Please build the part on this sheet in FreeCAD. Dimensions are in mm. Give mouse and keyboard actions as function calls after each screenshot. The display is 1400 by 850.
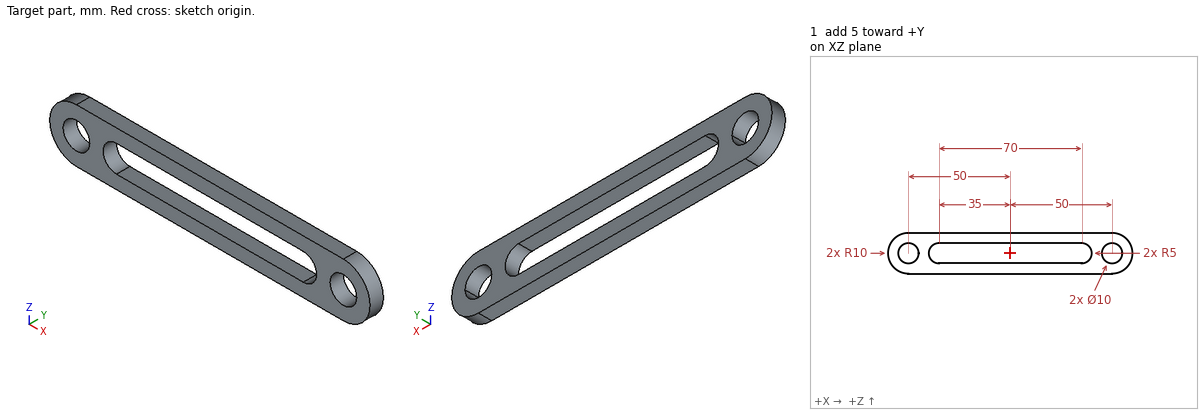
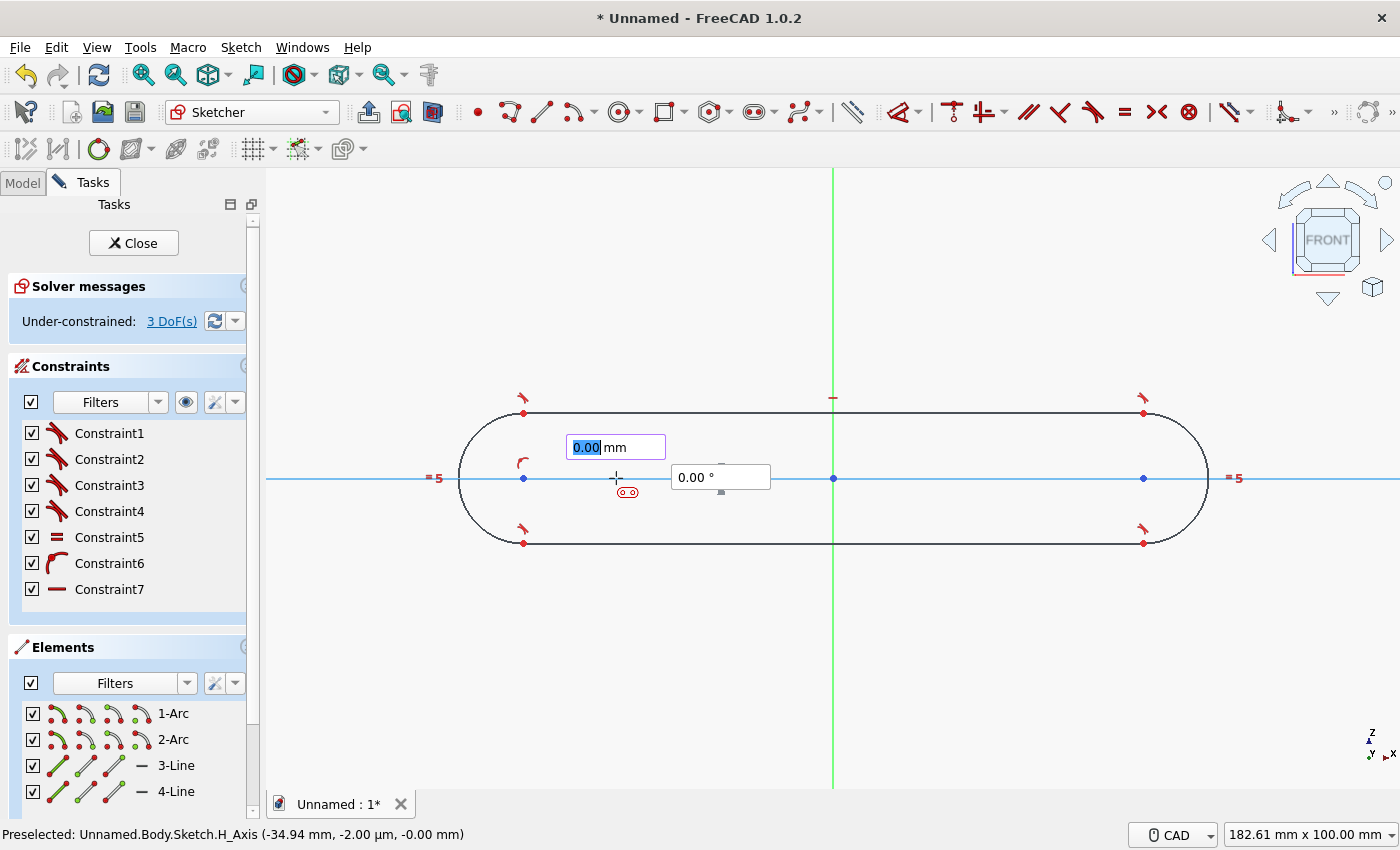
click(1050, 470)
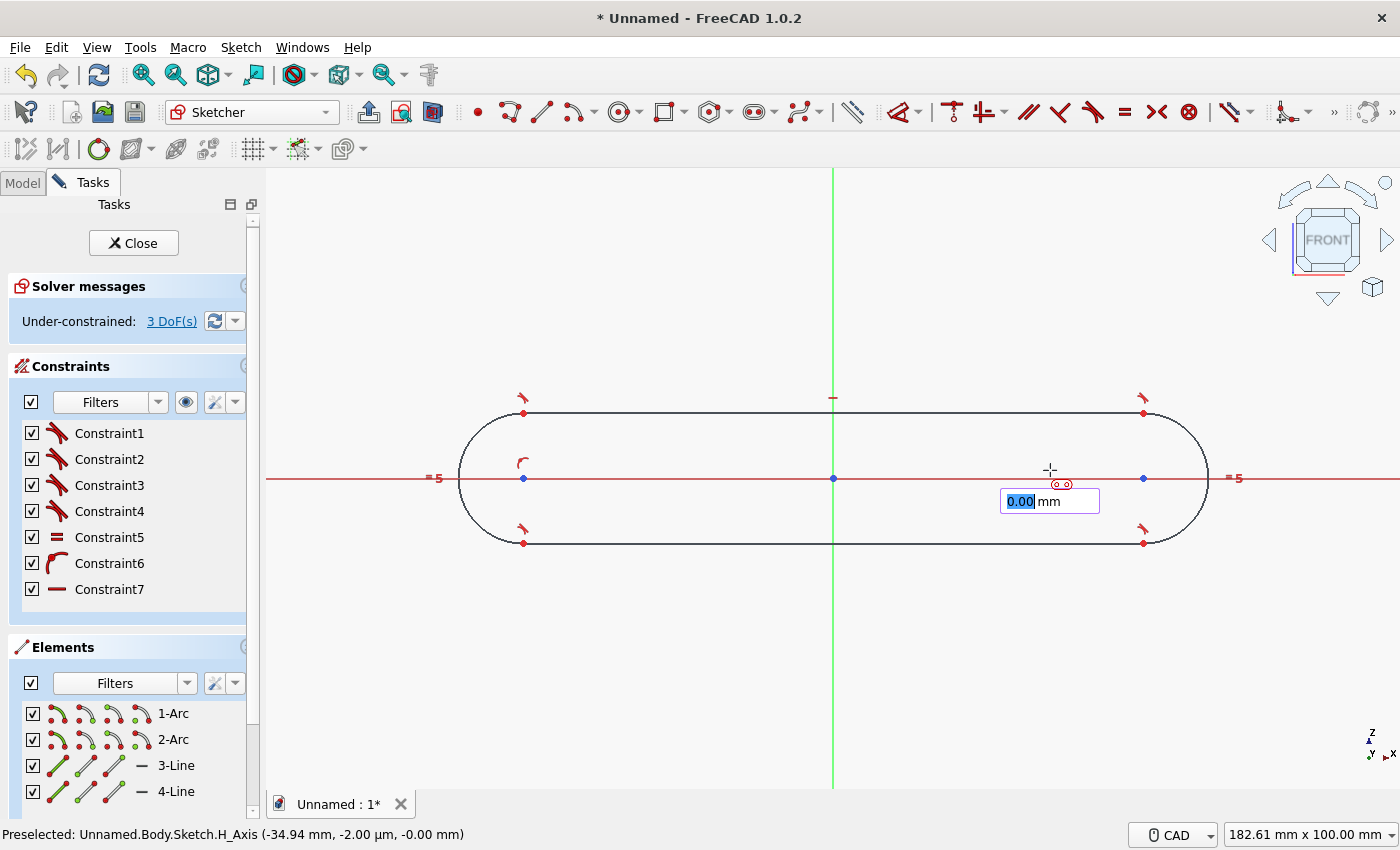
click(768, 510)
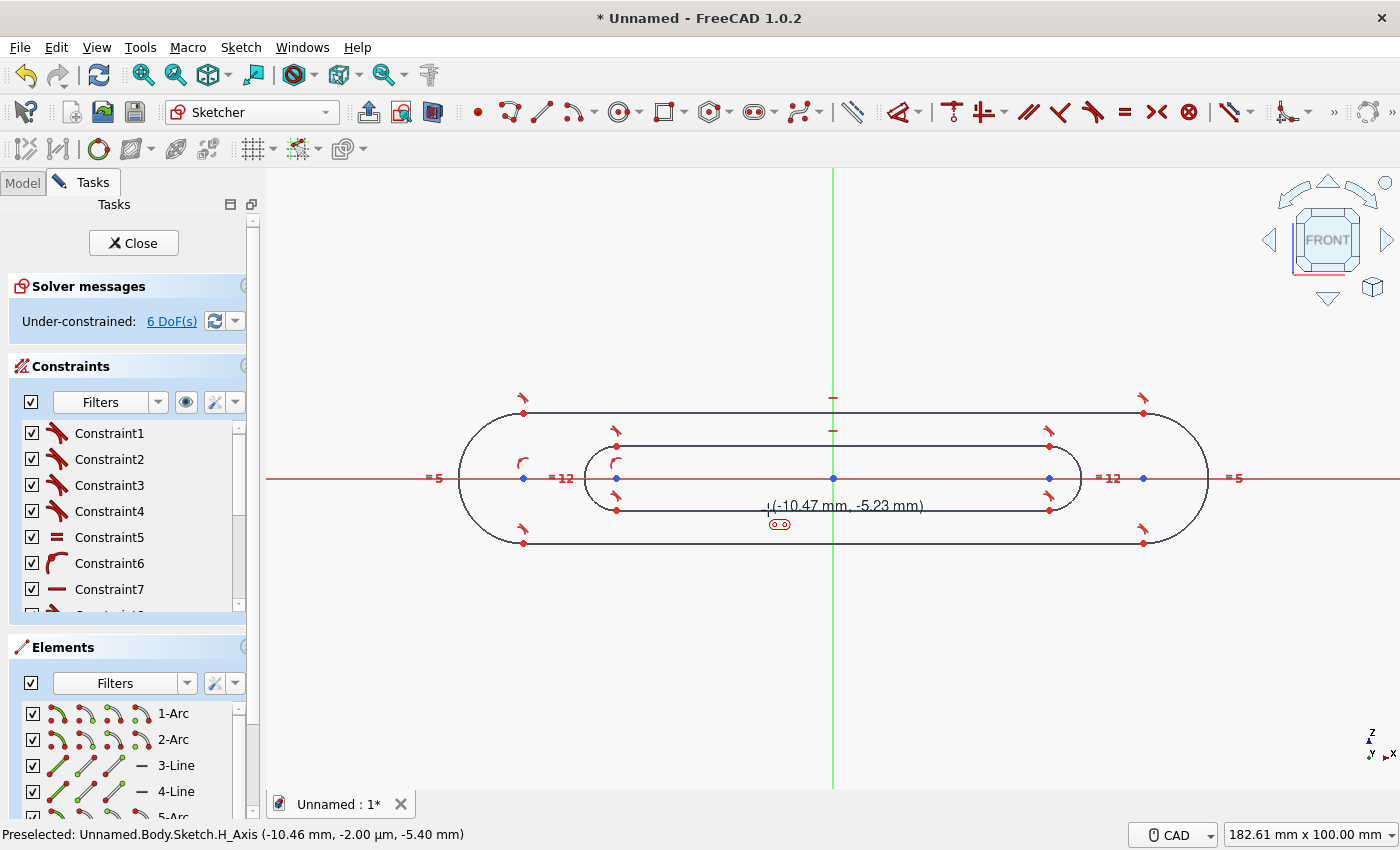
key(g)
key(c)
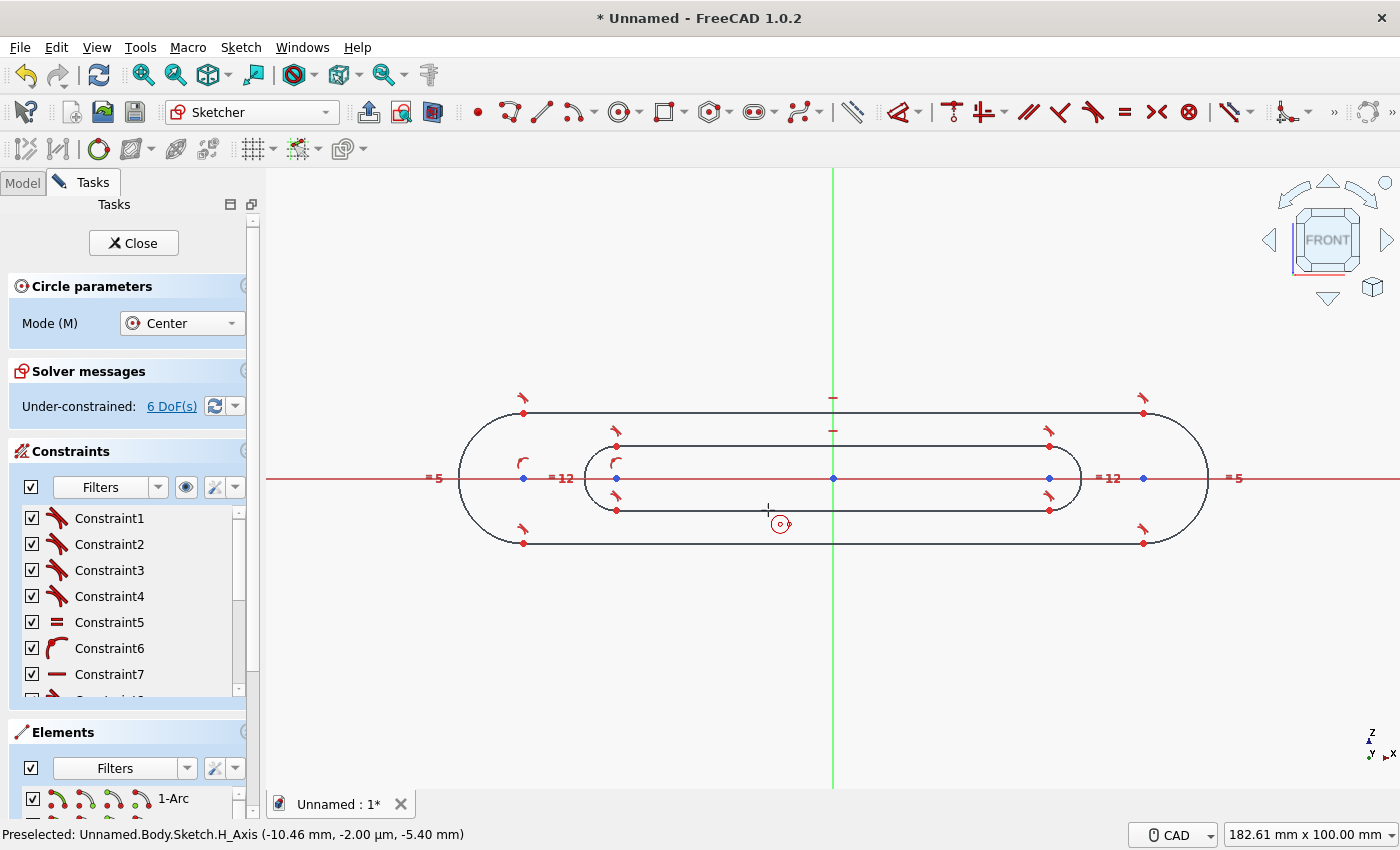
click(1143, 478)
click(1165, 457)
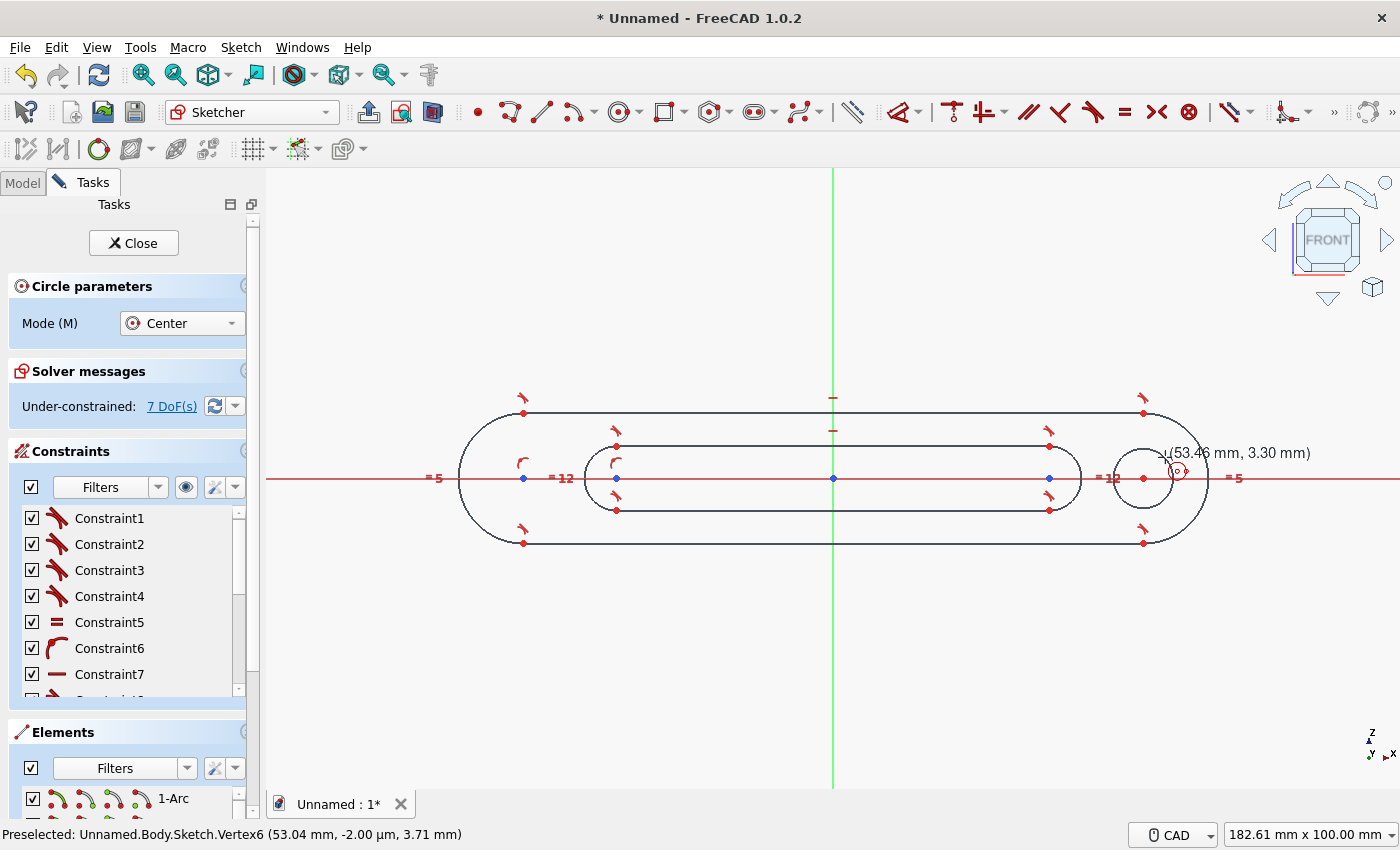
click(524, 478)
click(544, 457)
key(Escape)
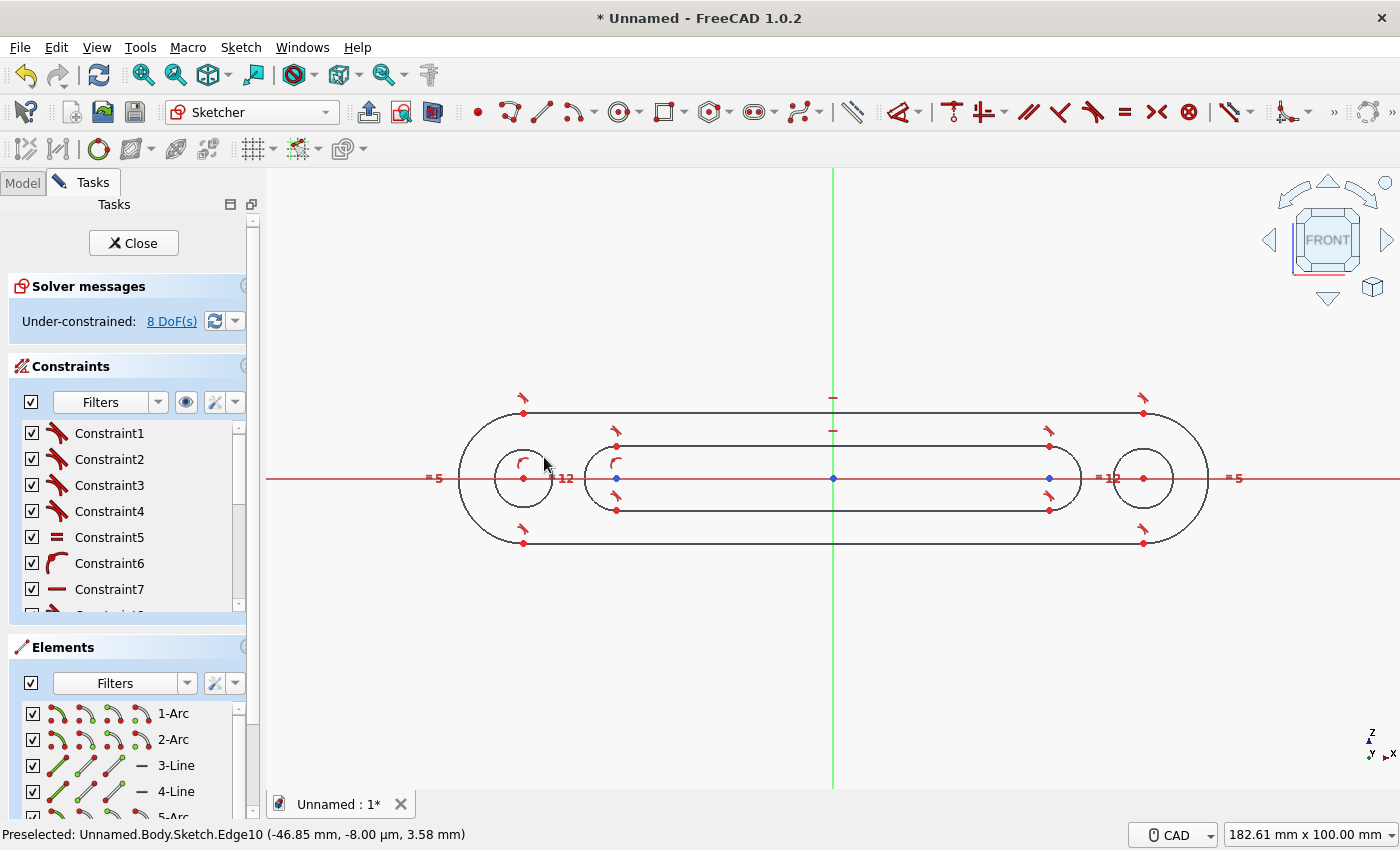
click(1164, 457)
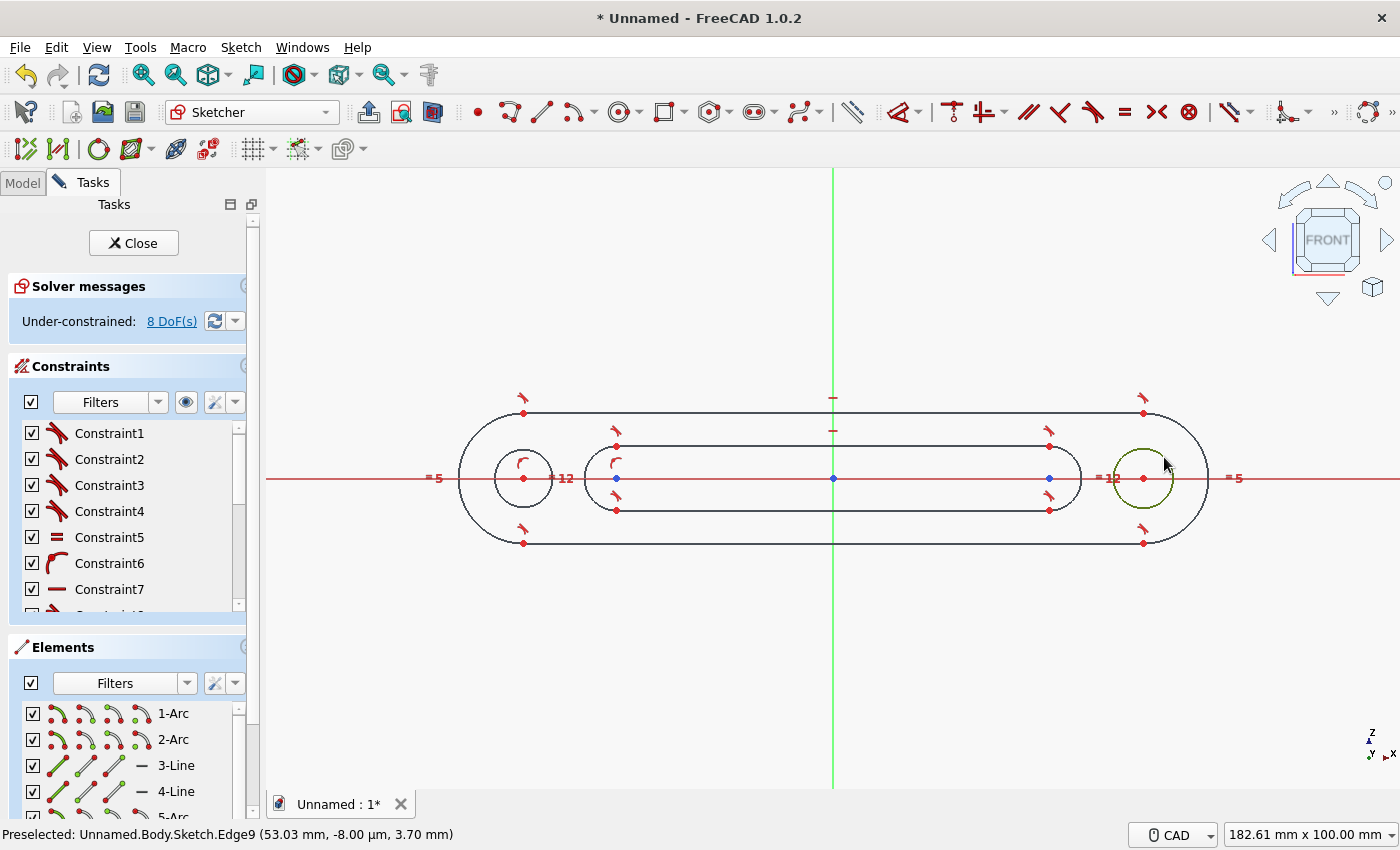
click(544, 458)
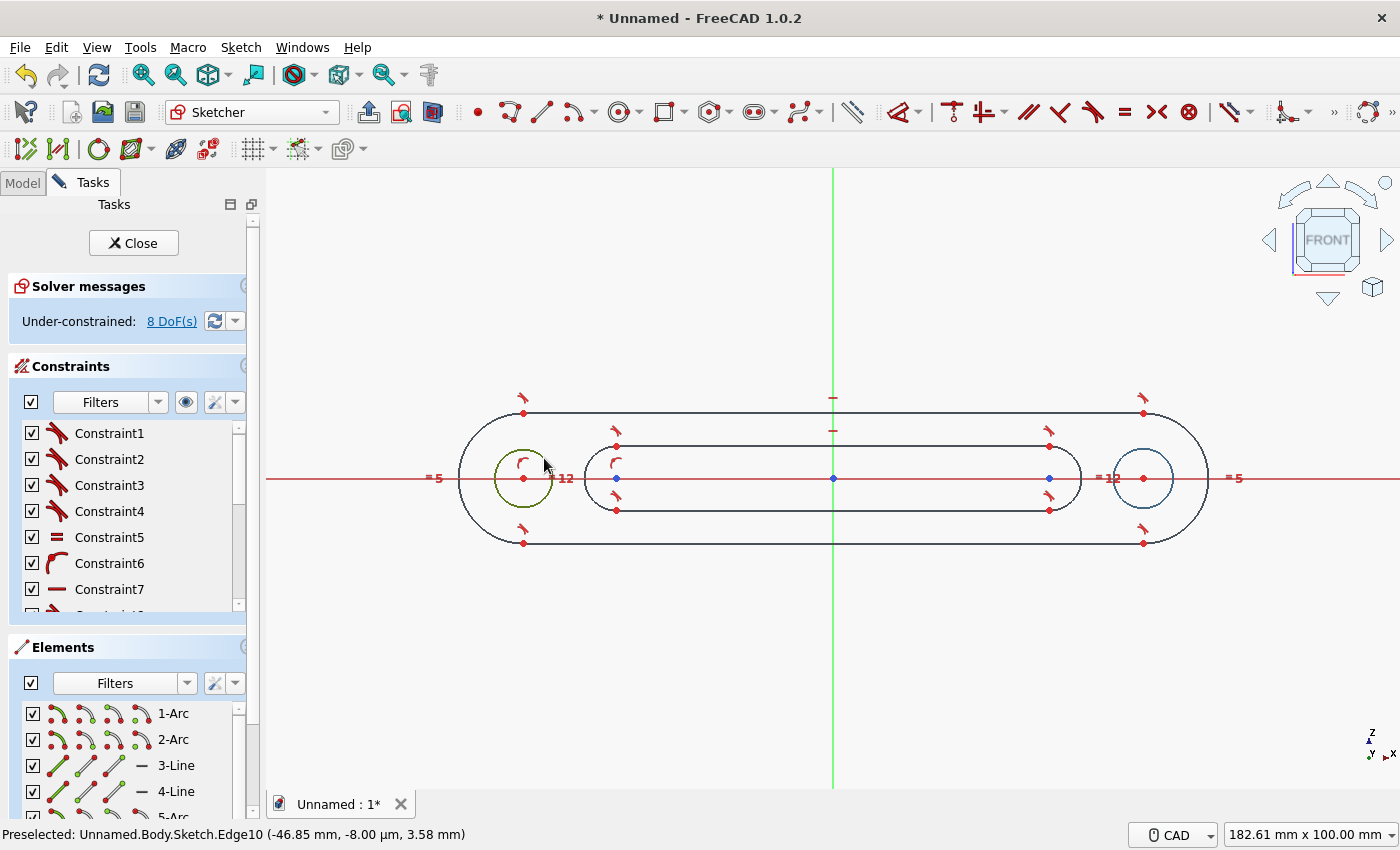
key(e)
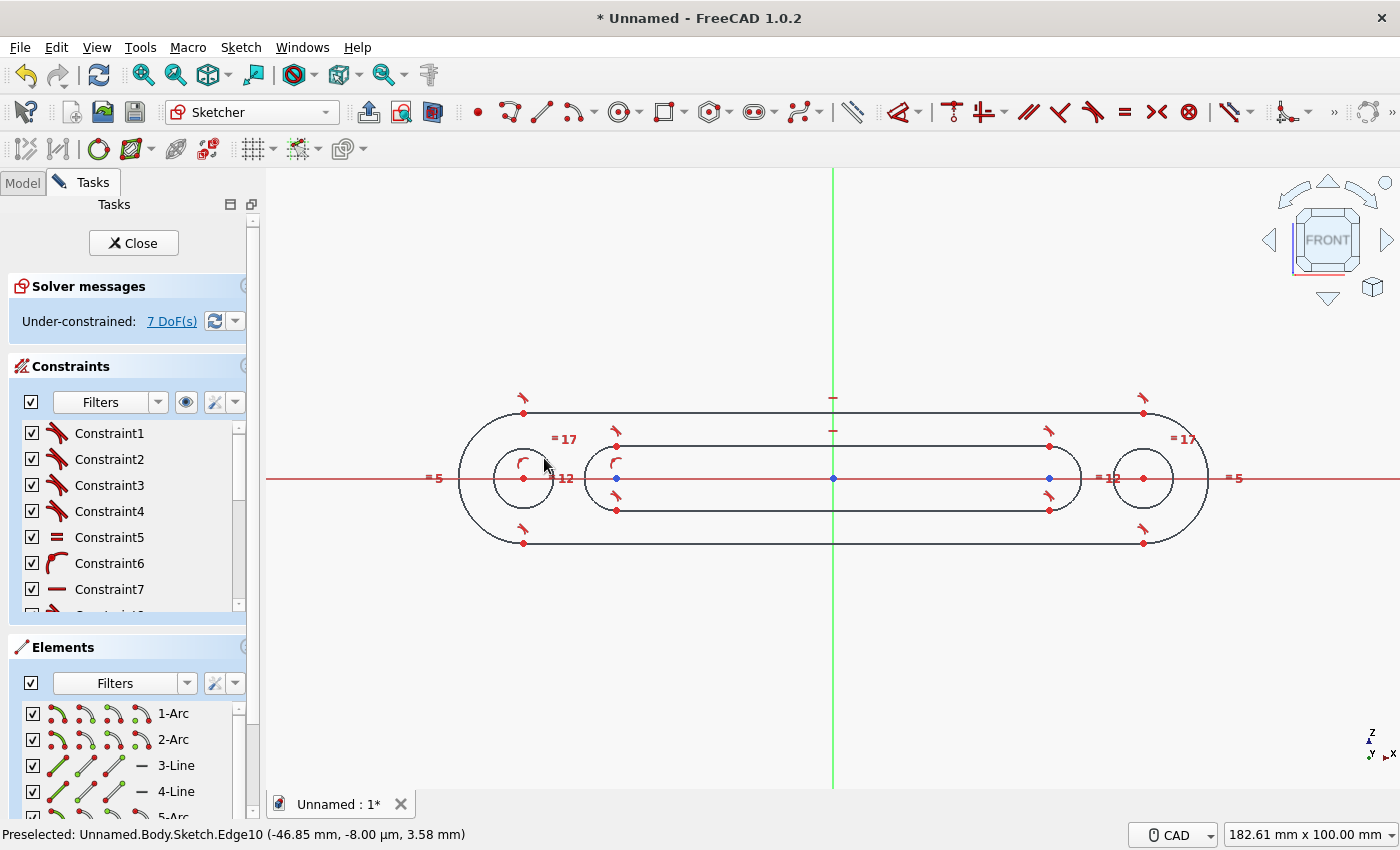
click(898, 112)